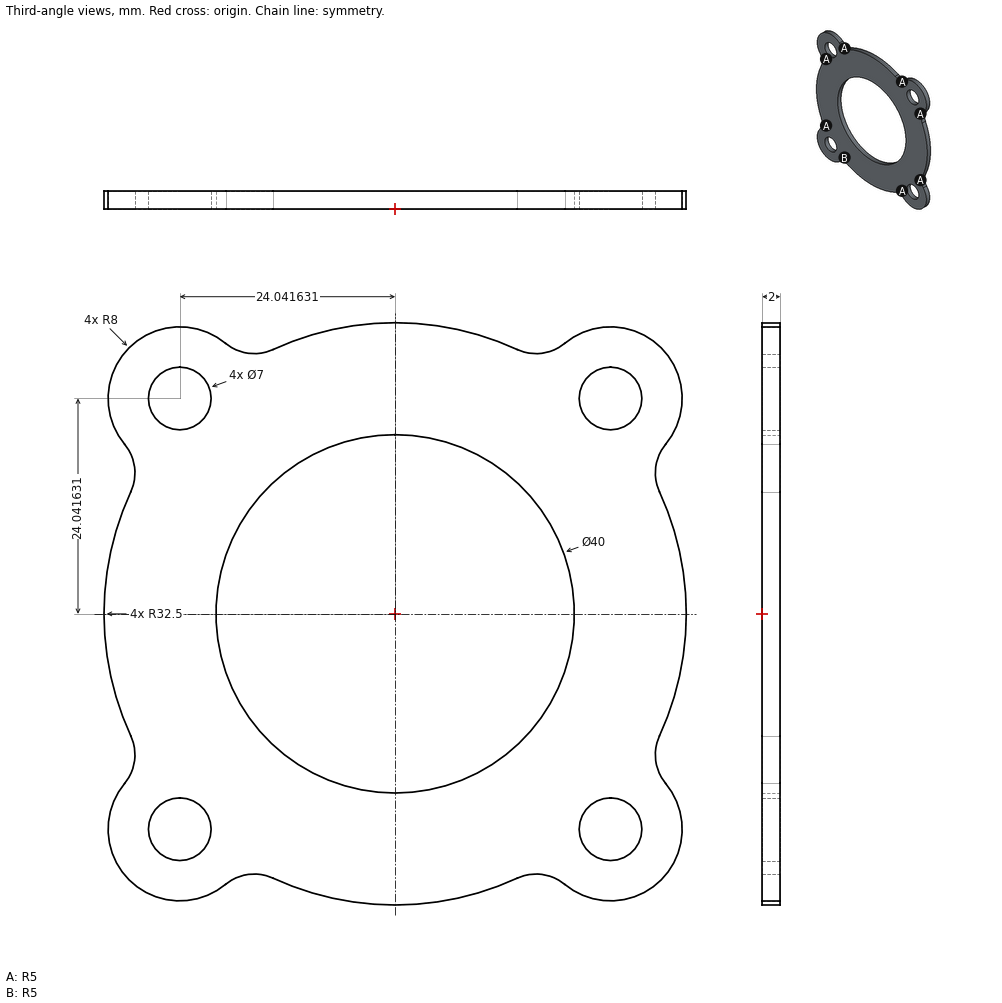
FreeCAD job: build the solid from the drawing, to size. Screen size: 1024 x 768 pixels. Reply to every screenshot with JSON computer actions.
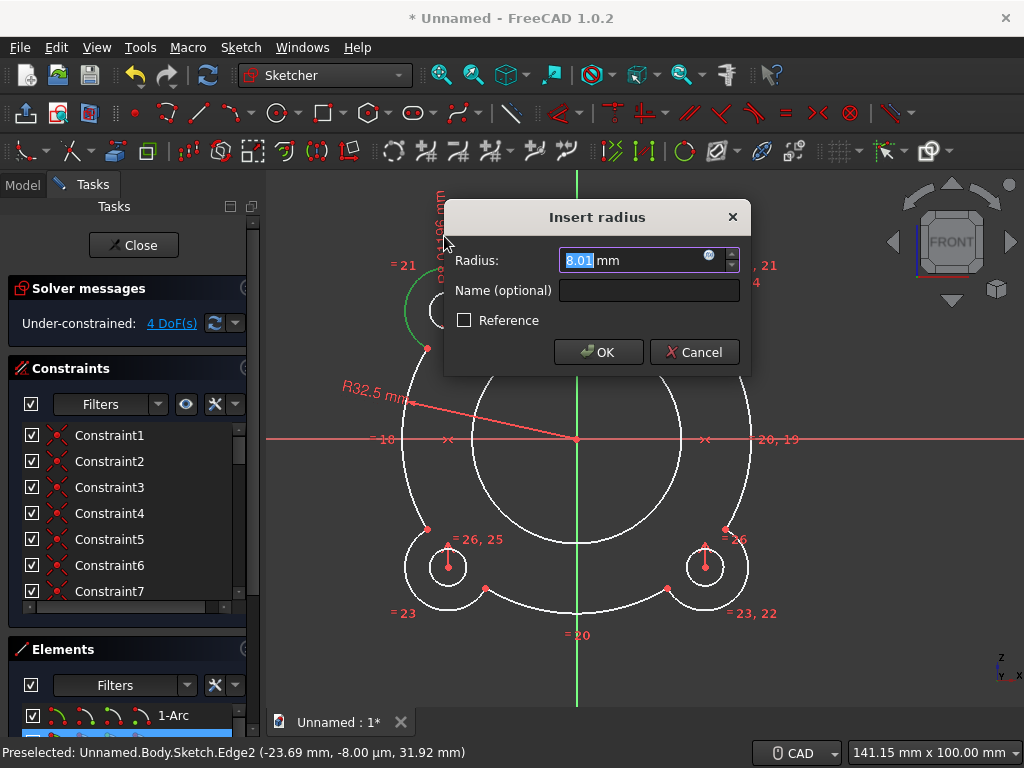
{"action": "type", "text": "8"}
{"action": "key", "text": "Return"}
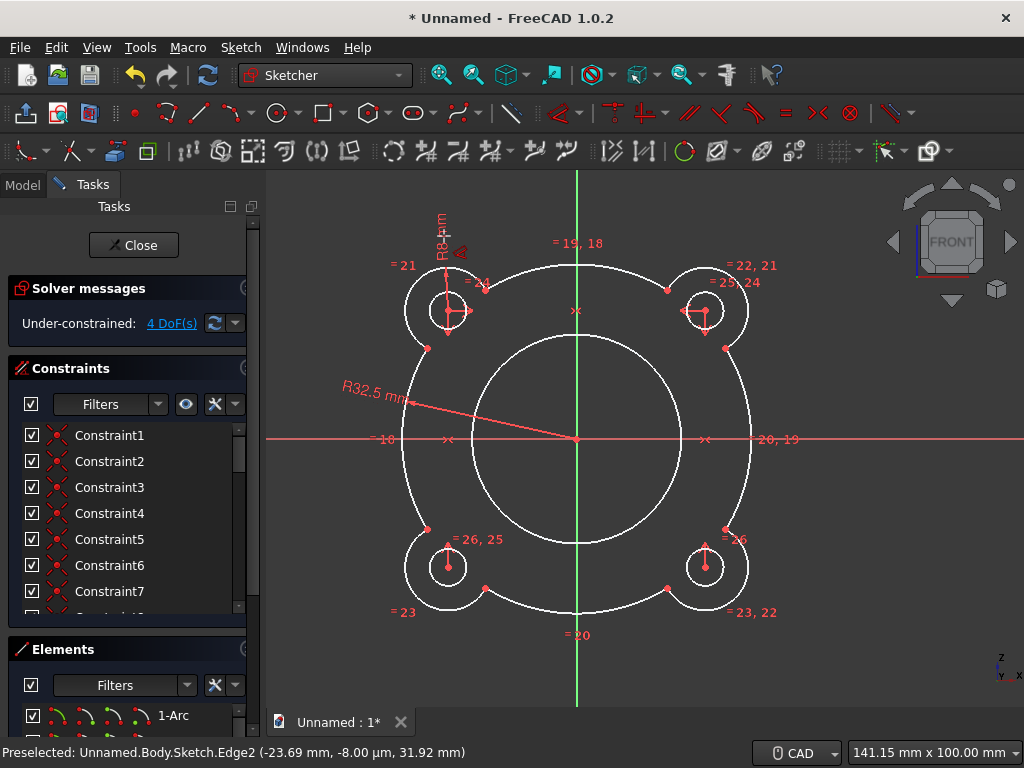
{"action": "left_click", "coordinate": [461, 298]}
{"action": "left_click", "coordinate": [497, 322]}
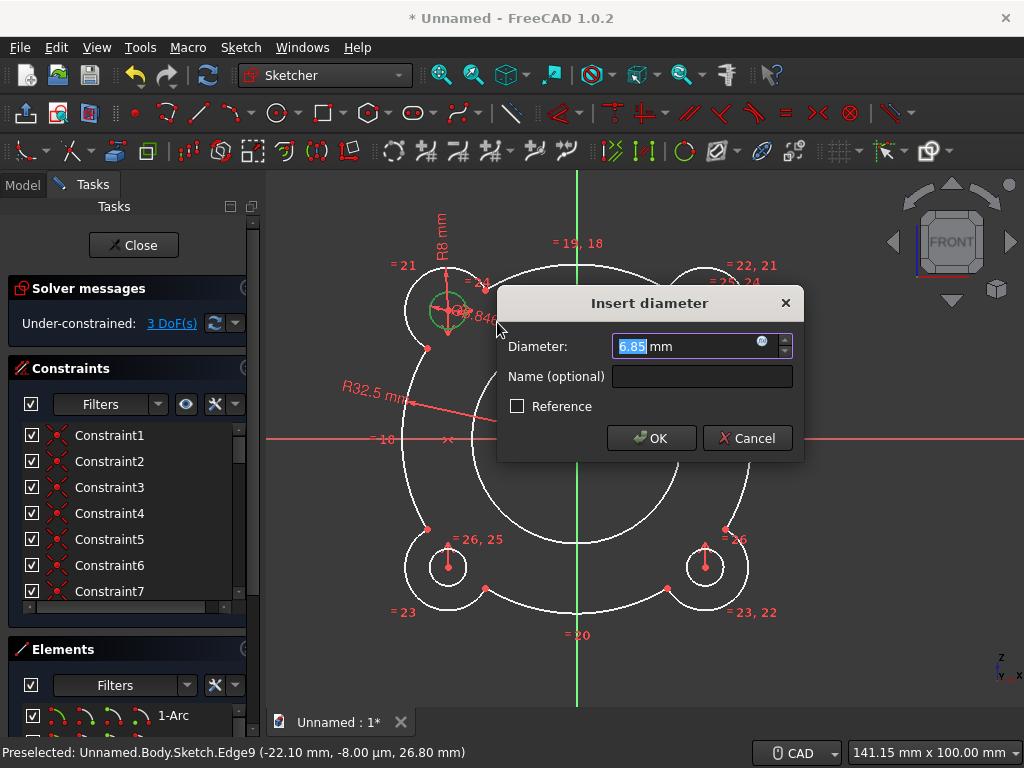
{"action": "type", "text": "7"}
{"action": "key", "text": "Return"}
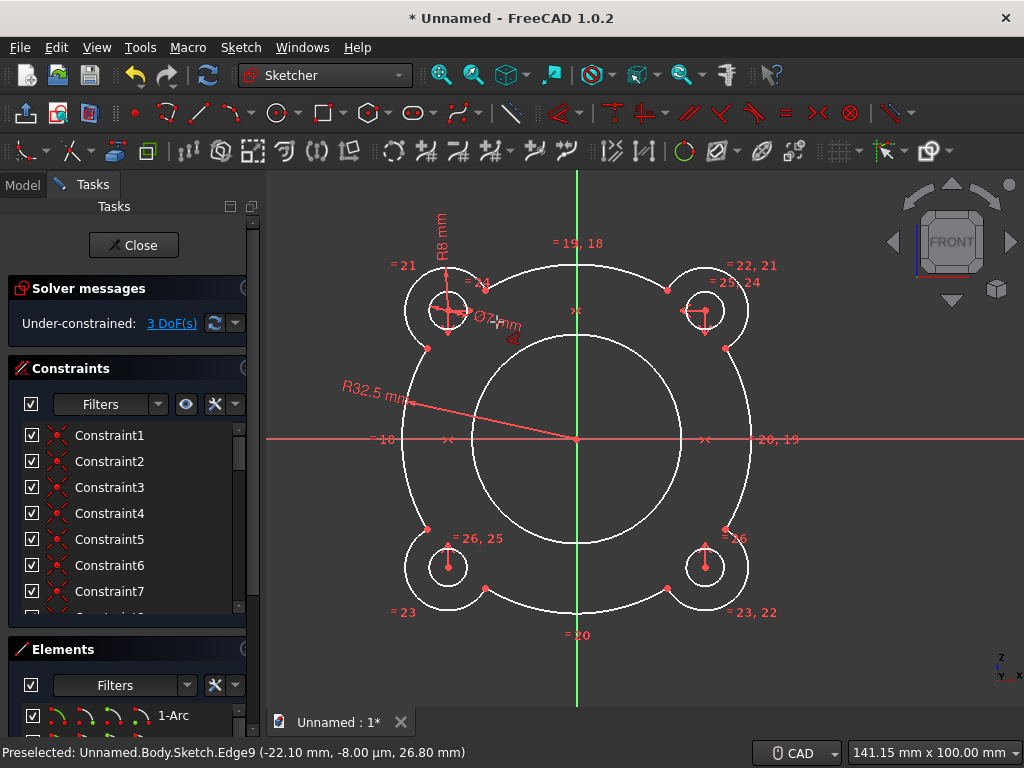
{"action": "left_click", "coordinate": [650, 365]}
{"action": "left_click", "coordinate": [673, 342]}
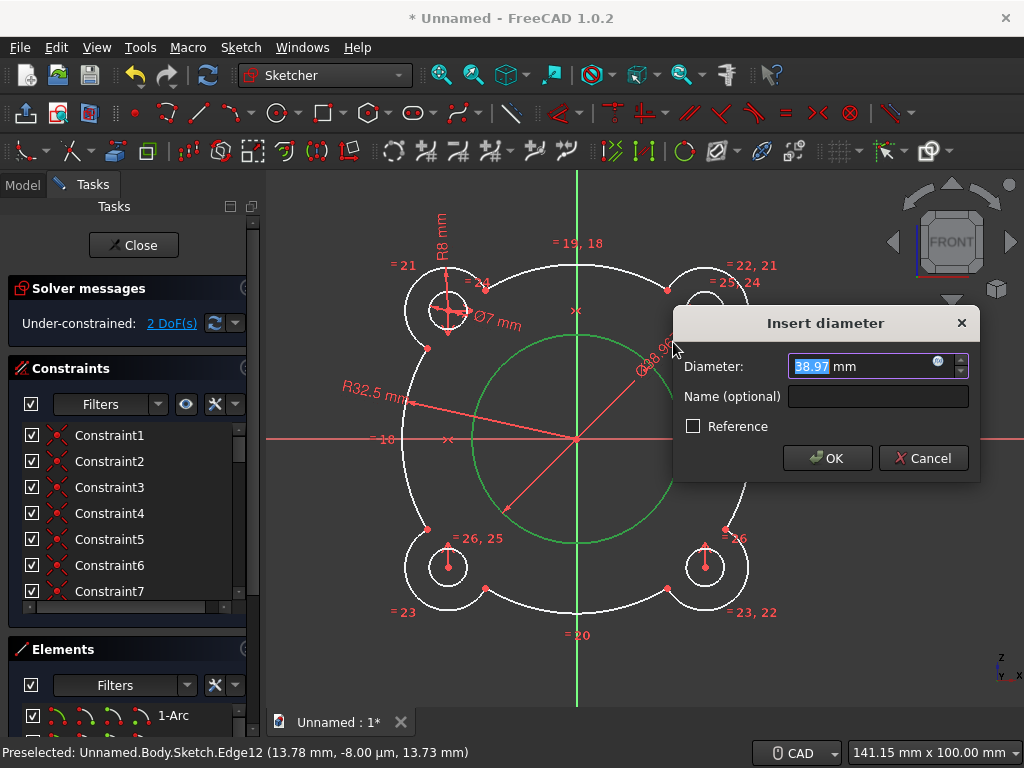
{"action": "type", "text": "40"}
{"action": "key", "text": "Return"}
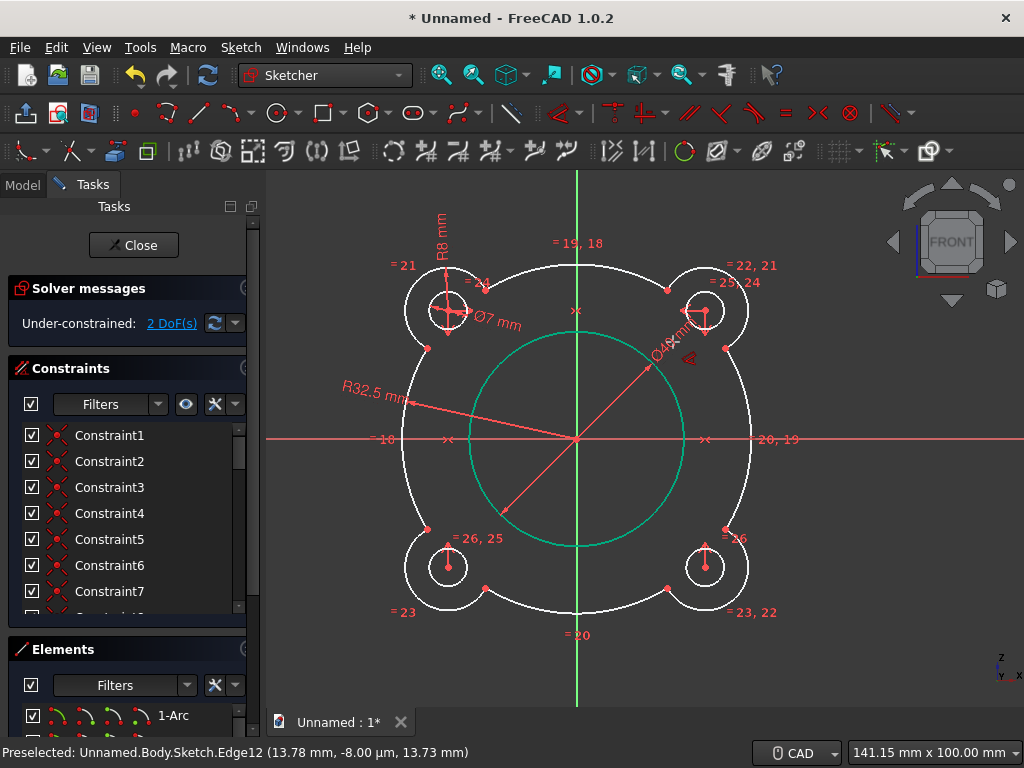
{"action": "left_click", "coordinate": [448, 311]}
{"action": "left_click", "coordinate": [512, 473]}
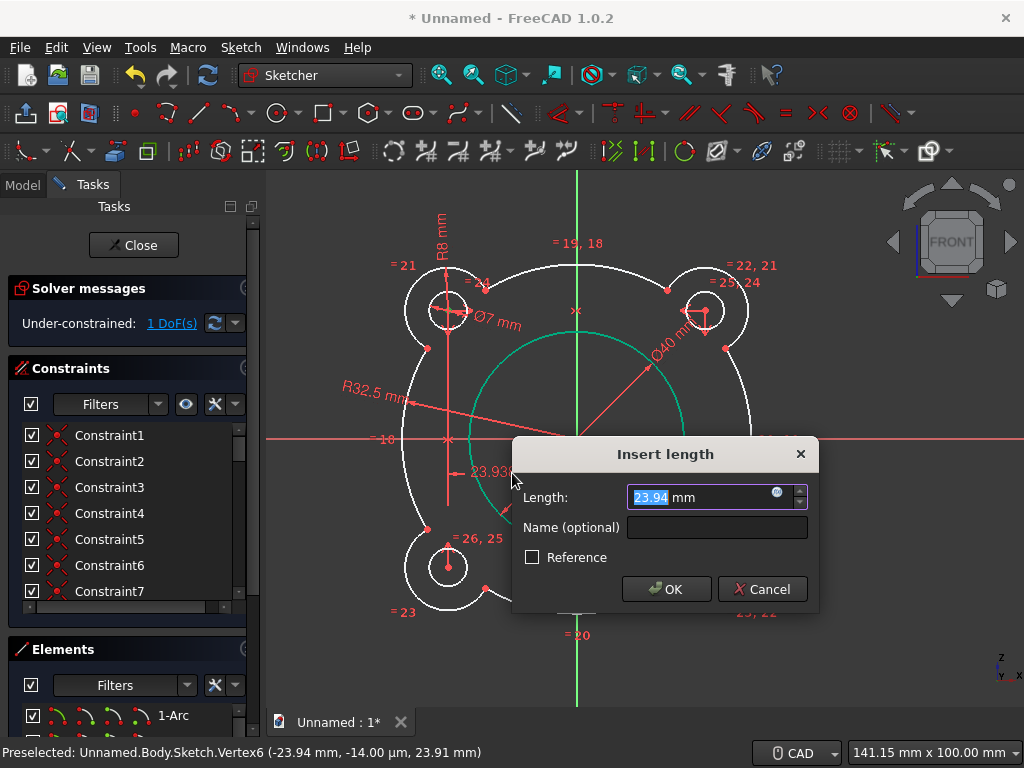
{"action": "type", "text": "24.041631"}
{"action": "key", "text": "Return"}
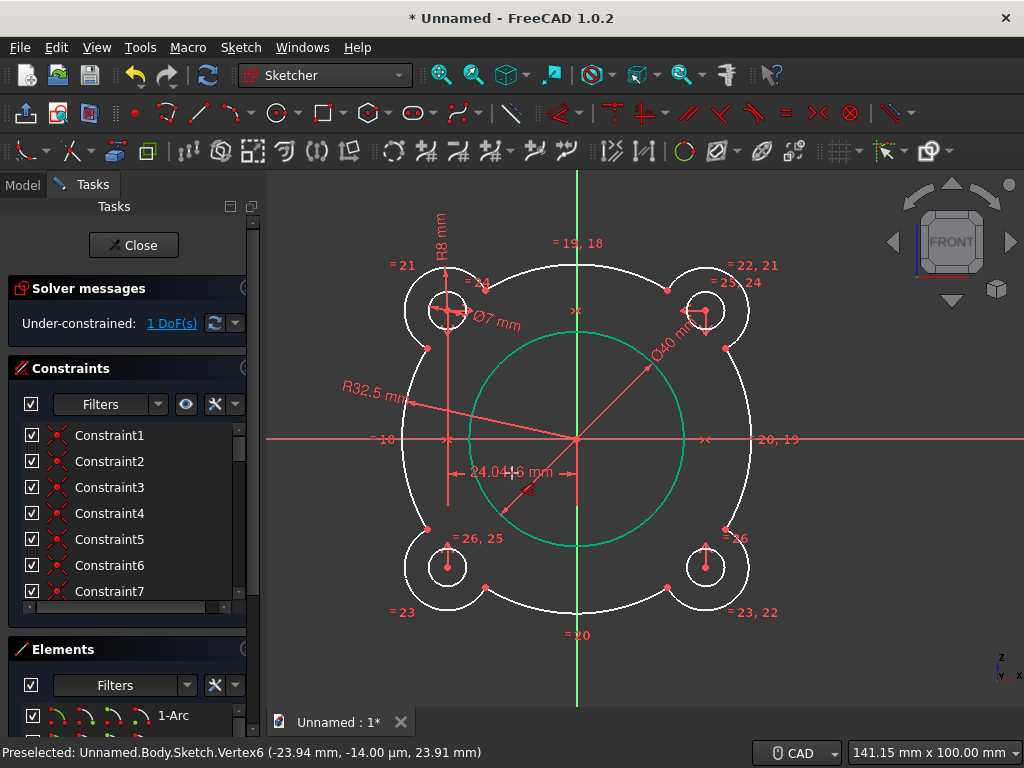
{"action": "left_click", "coordinate": [448, 311]}
{"action": "left_click", "coordinate": [611, 375]}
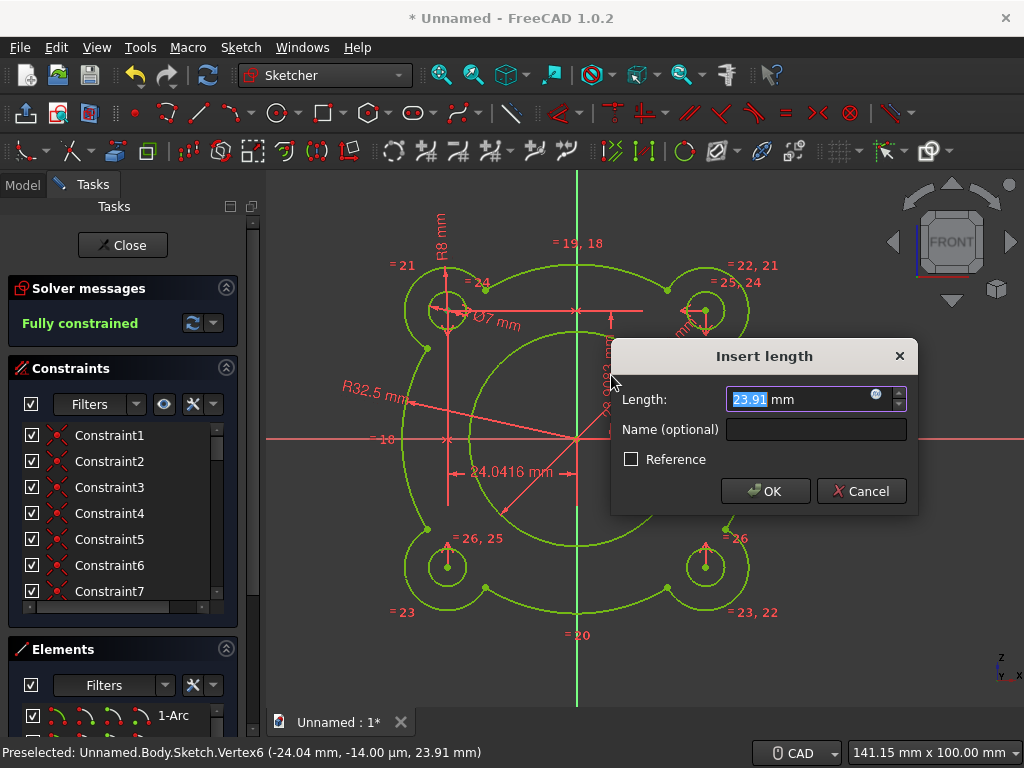
{"action": "type", "text": "24.041631"}
{"action": "key", "text": "Return"}
{"action": "key", "text": "Escape"}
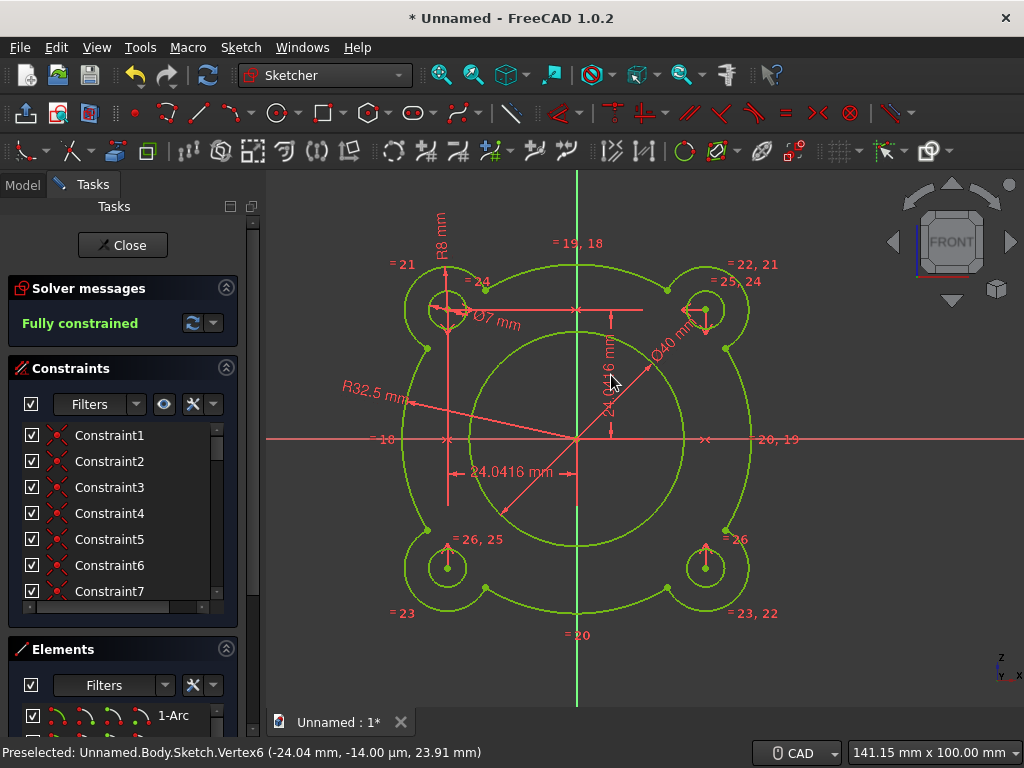
{"action": "left_click", "coordinate": [123, 245]}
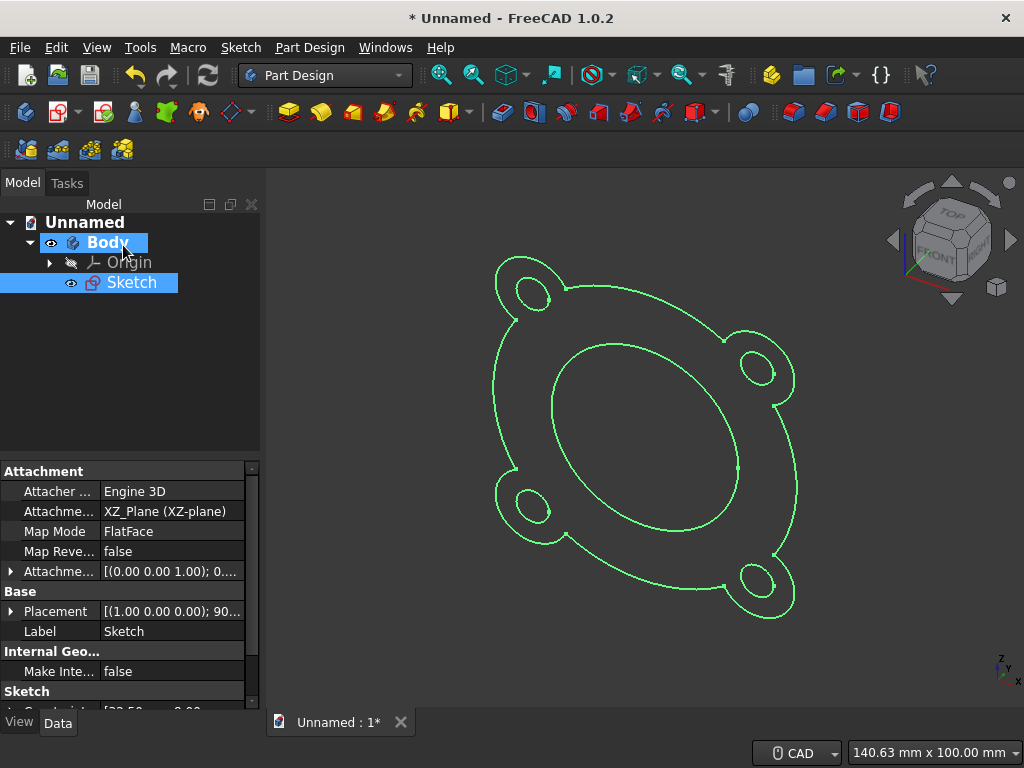
{"action": "left_click", "coordinate": [290, 112]}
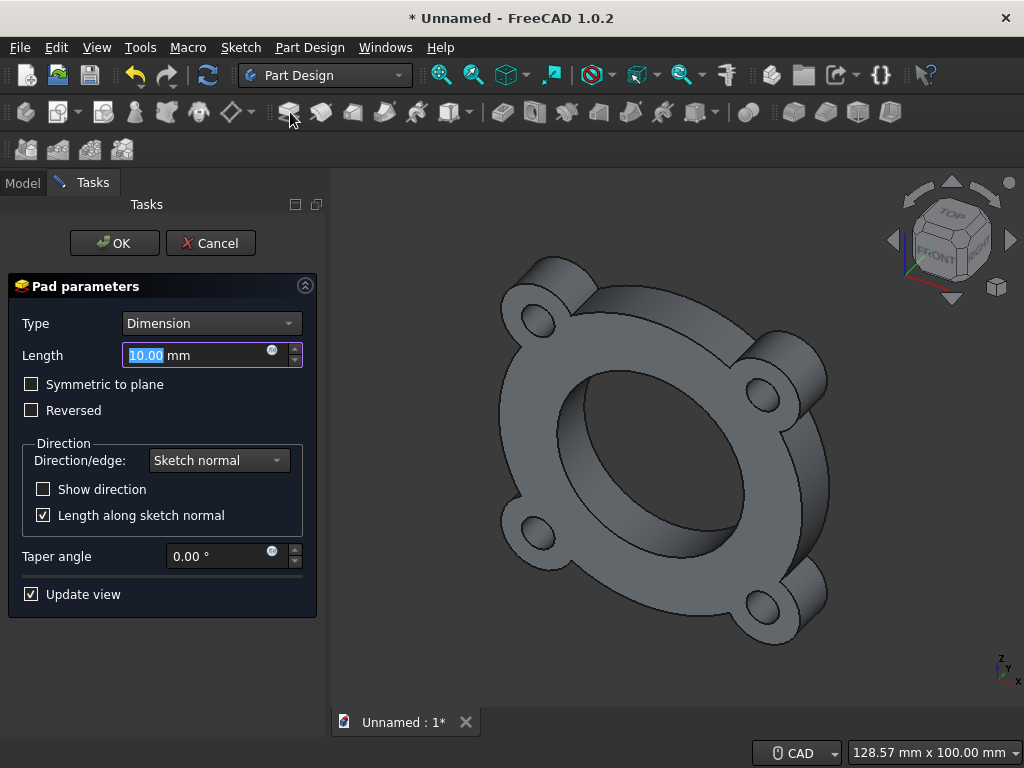
{"action": "type", "text": "2"}
{"action": "key", "text": "Tab"}